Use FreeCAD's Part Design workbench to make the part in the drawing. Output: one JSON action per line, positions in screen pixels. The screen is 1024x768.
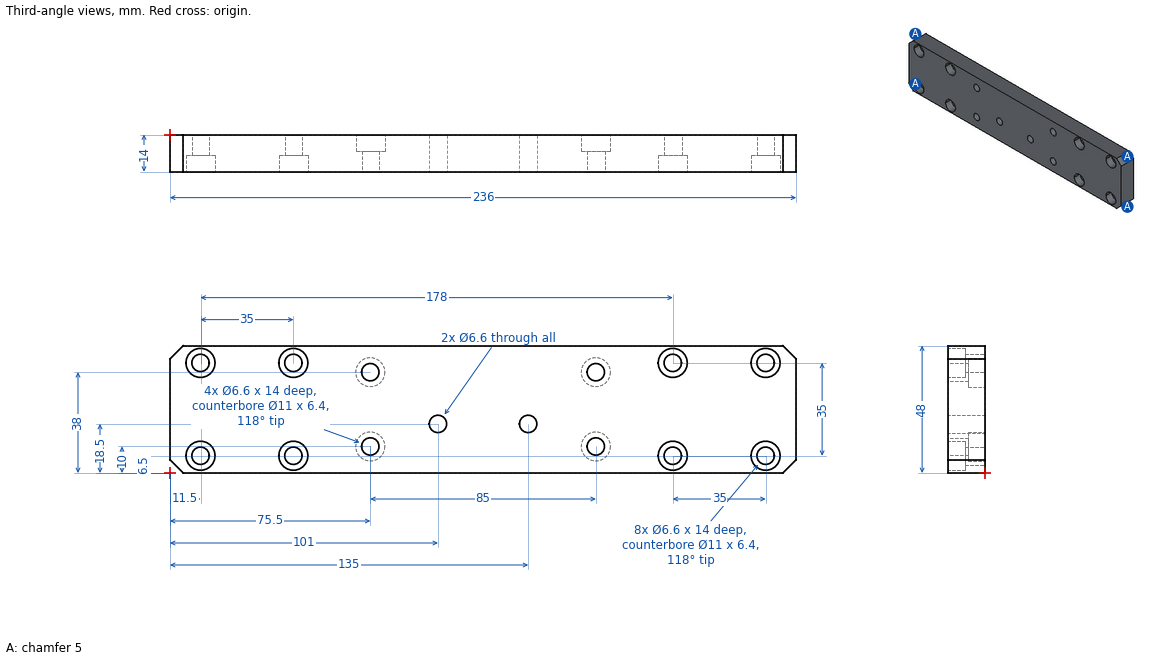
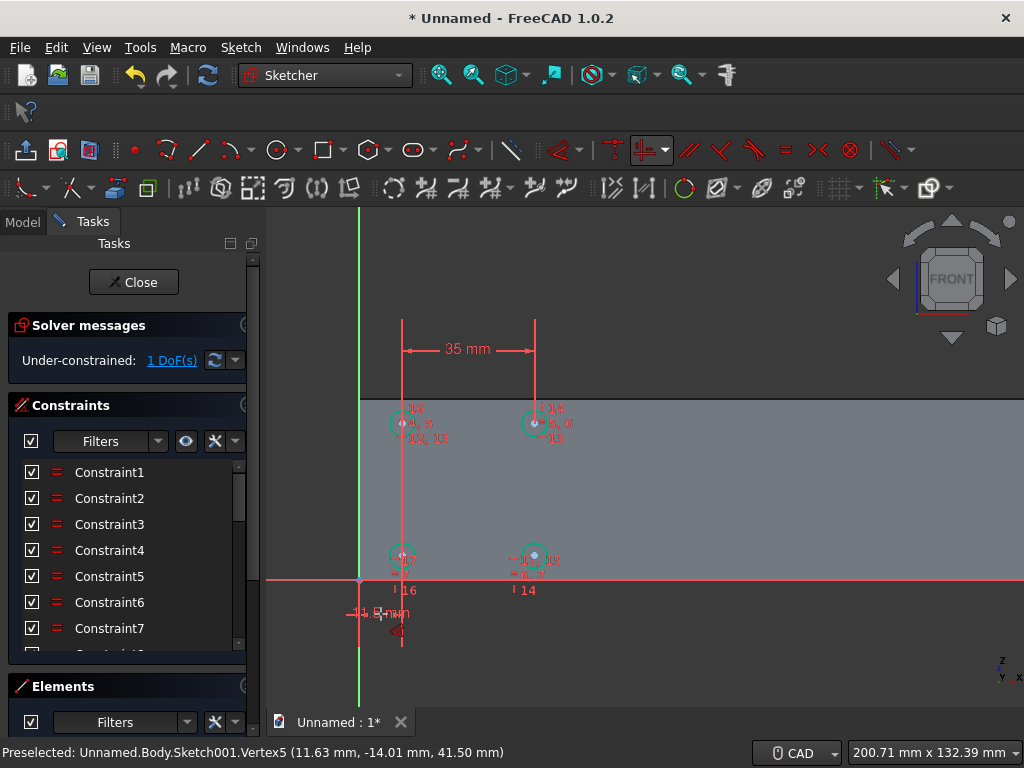
{"action": "scroll", "coordinate": [403, 425], "scroll_direction": "down", "scroll_amount": 4}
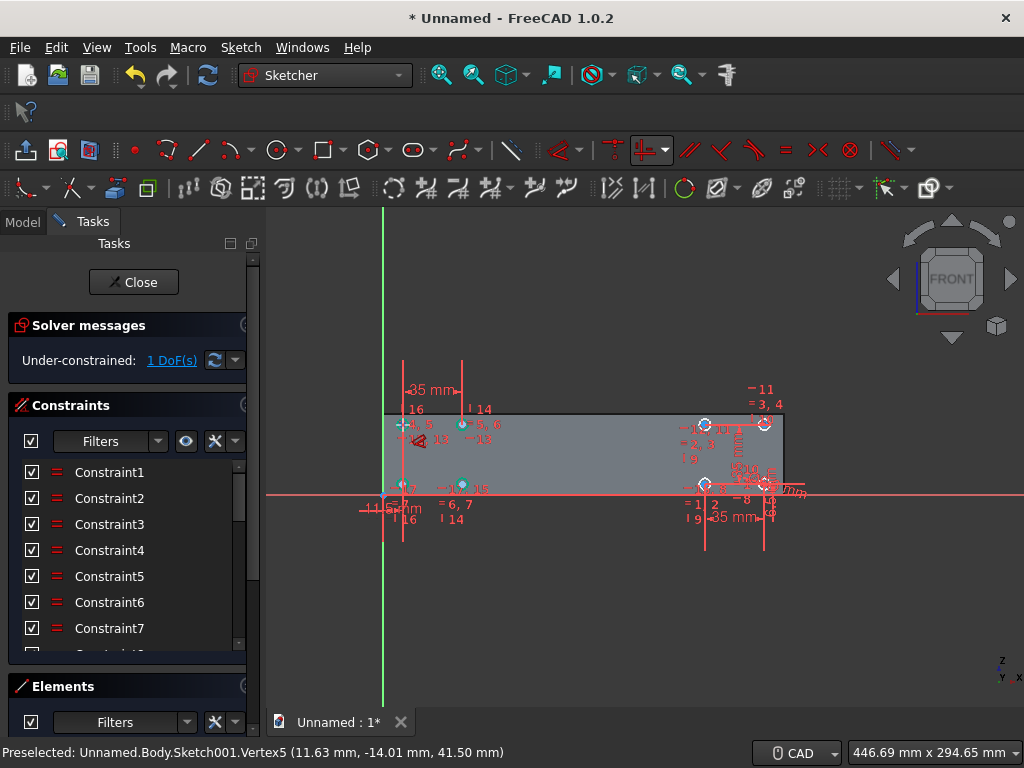
{"action": "left_click", "coordinate": [705, 425]}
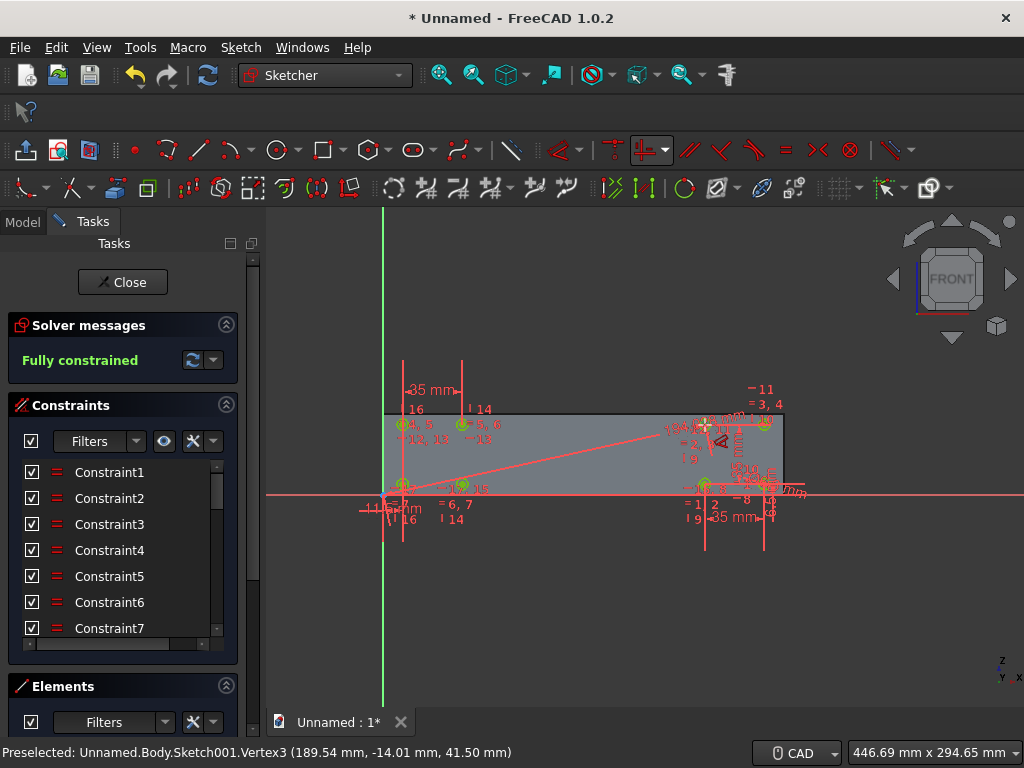
{"action": "left_click", "coordinate": [403, 425]}
{"action": "left_click", "coordinate": [554, 391]}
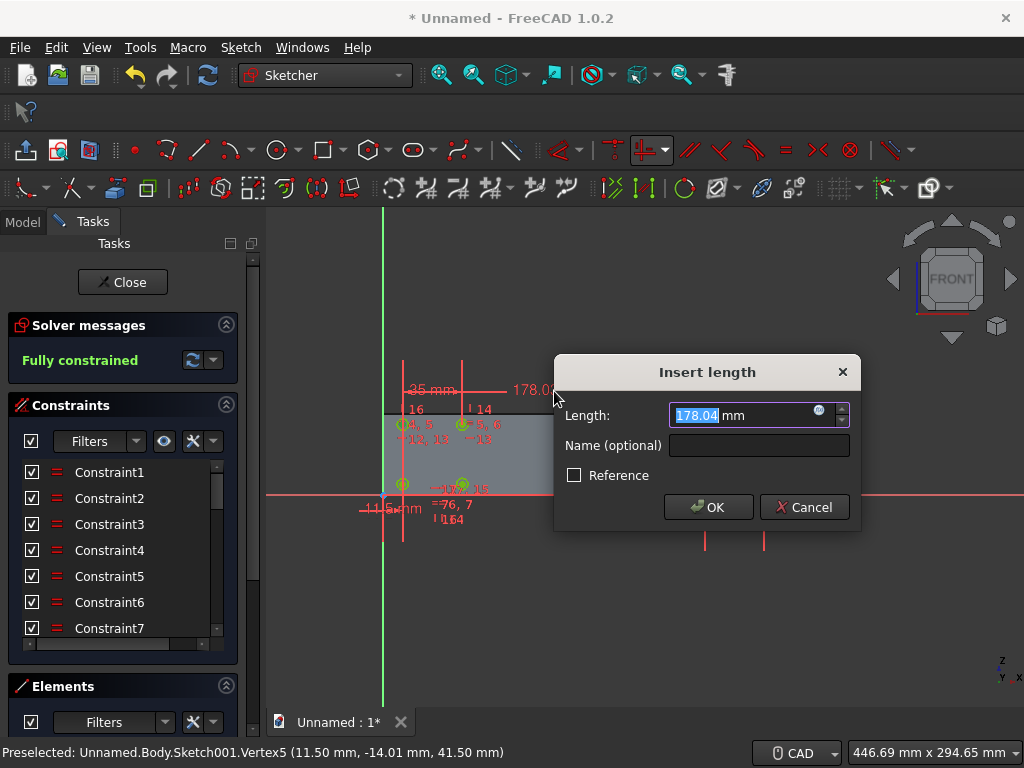
{"action": "type", "text": "178"}
{"action": "key", "text": "Return"}
{"action": "key", "text": "Escape"}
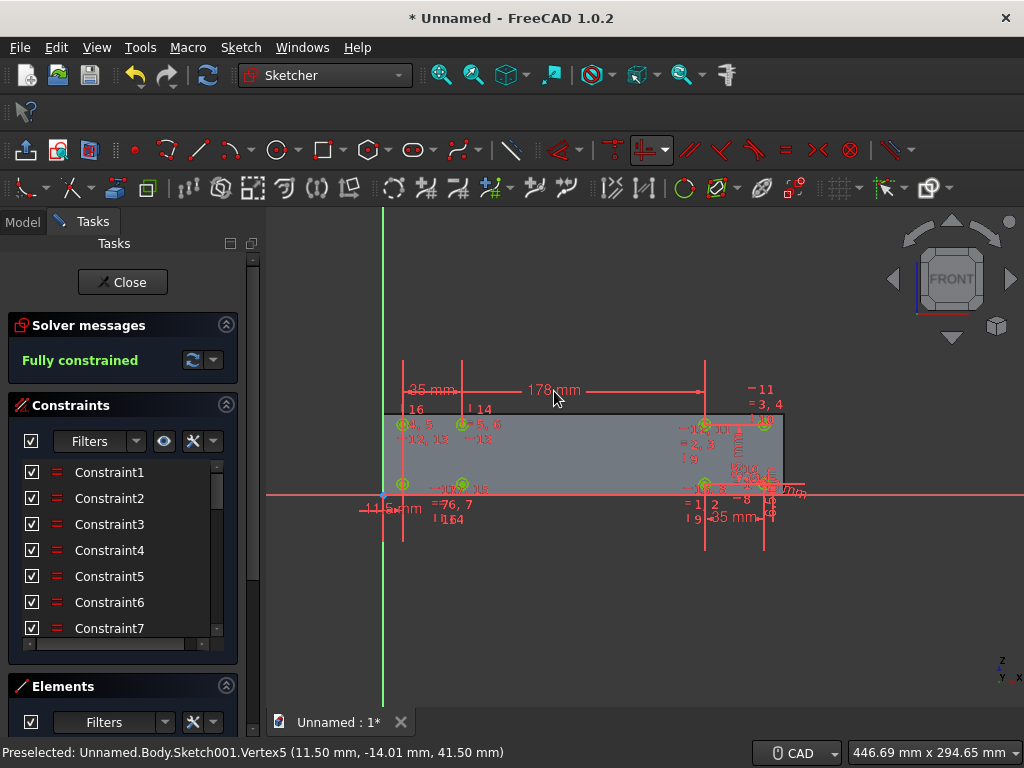
{"action": "left_click", "coordinate": [123, 282]}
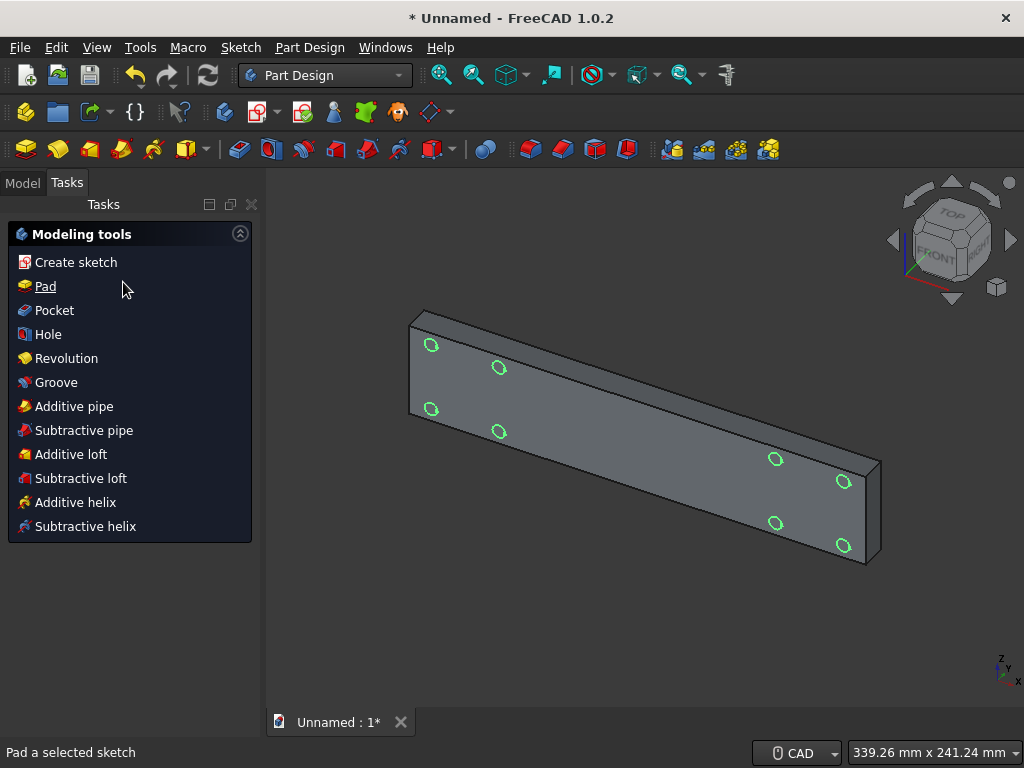
{"action": "left_click", "coordinate": [272, 150]}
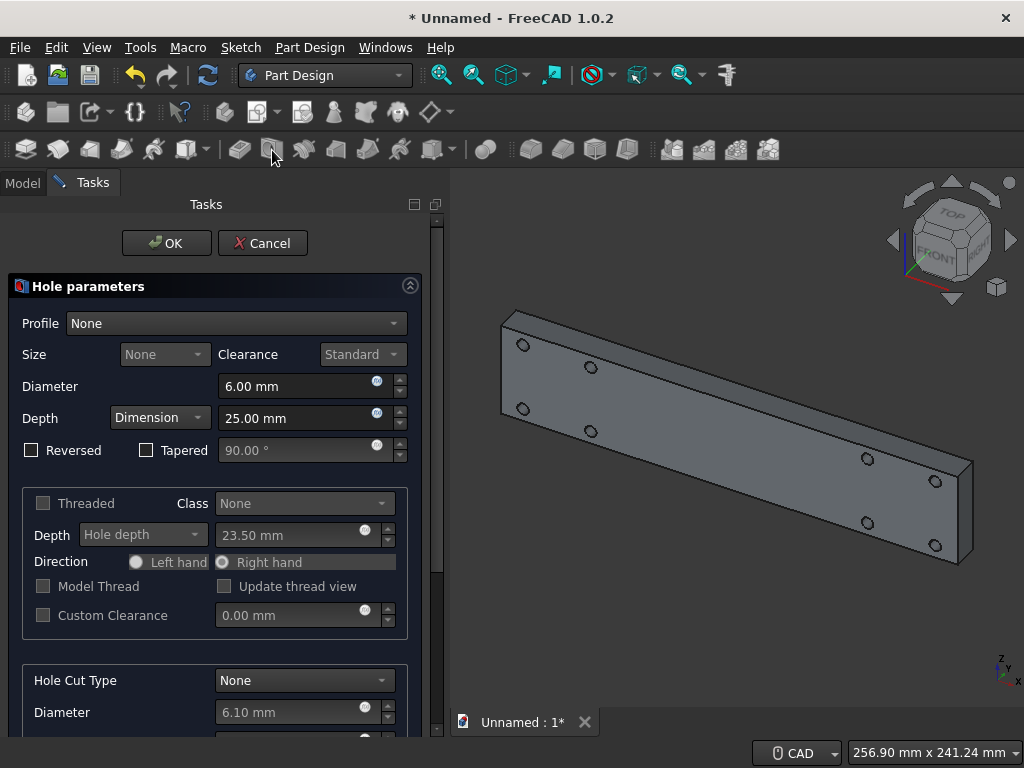
{"action": "triple_click", "coordinate": [305, 386]}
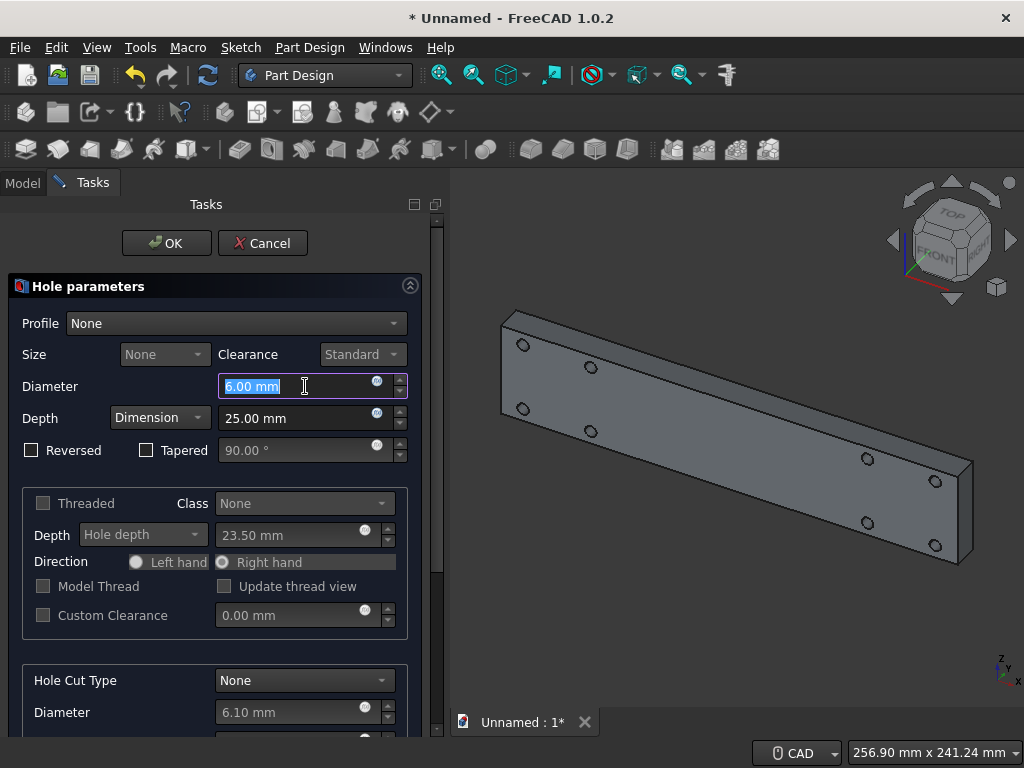
{"action": "type", "text": "6.6"}
{"action": "key", "text": "Tab"}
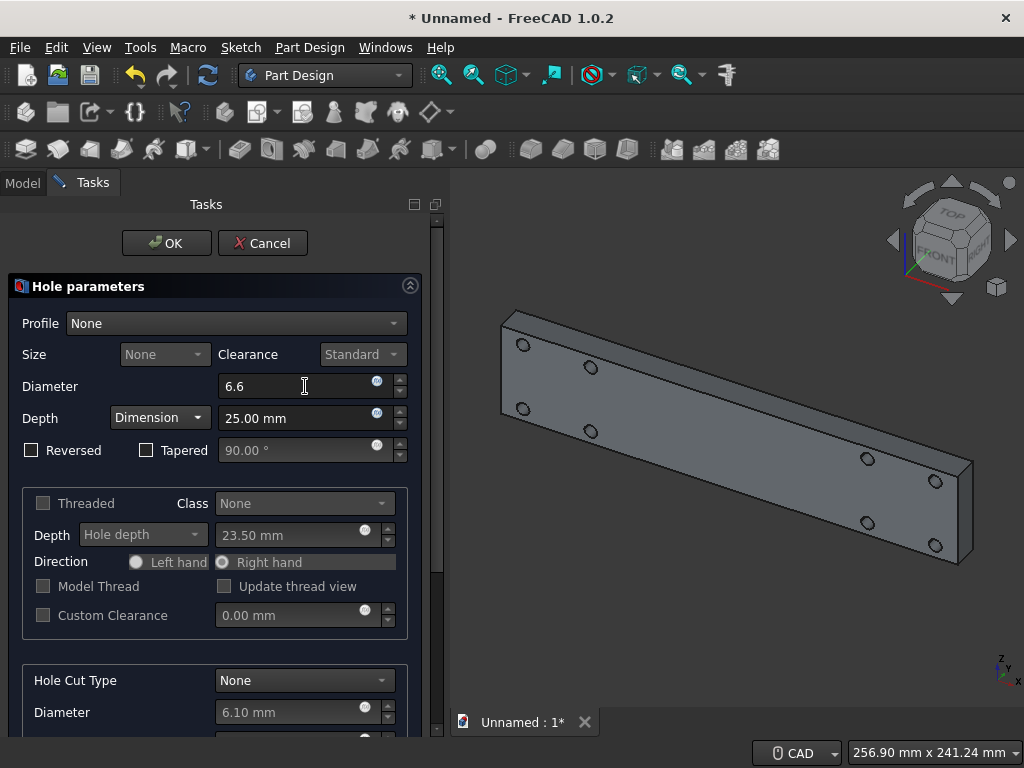
{"action": "triple_click", "coordinate": [305, 418]}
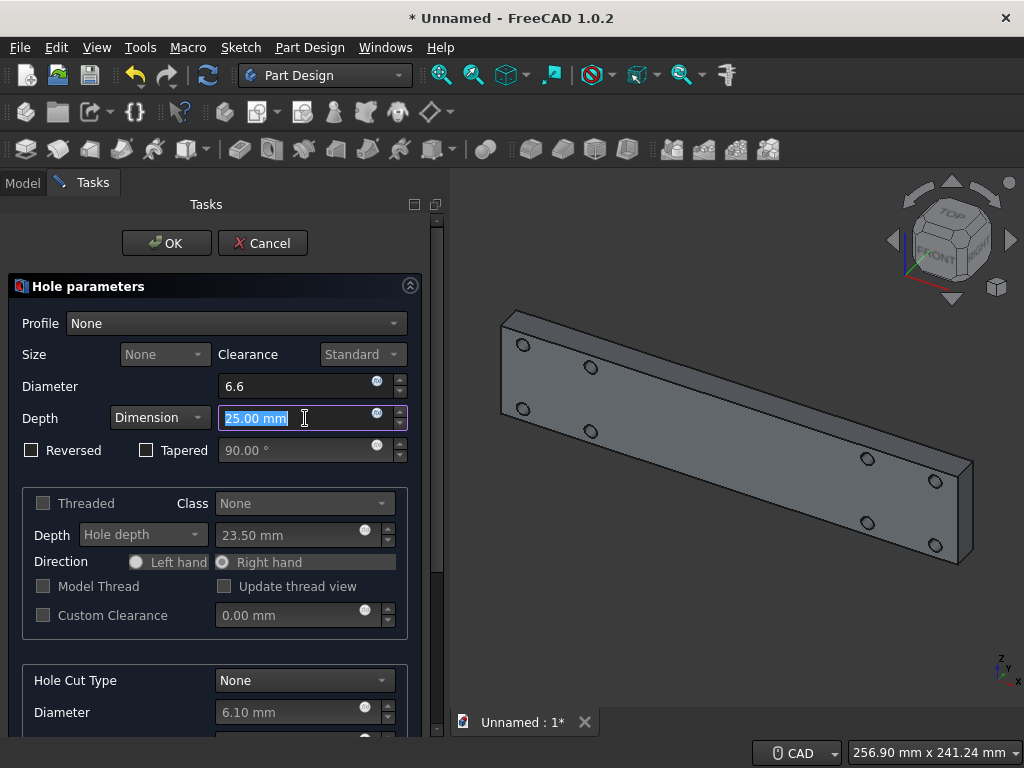
{"action": "type", "text": "14"}
{"action": "key", "text": "Tab"}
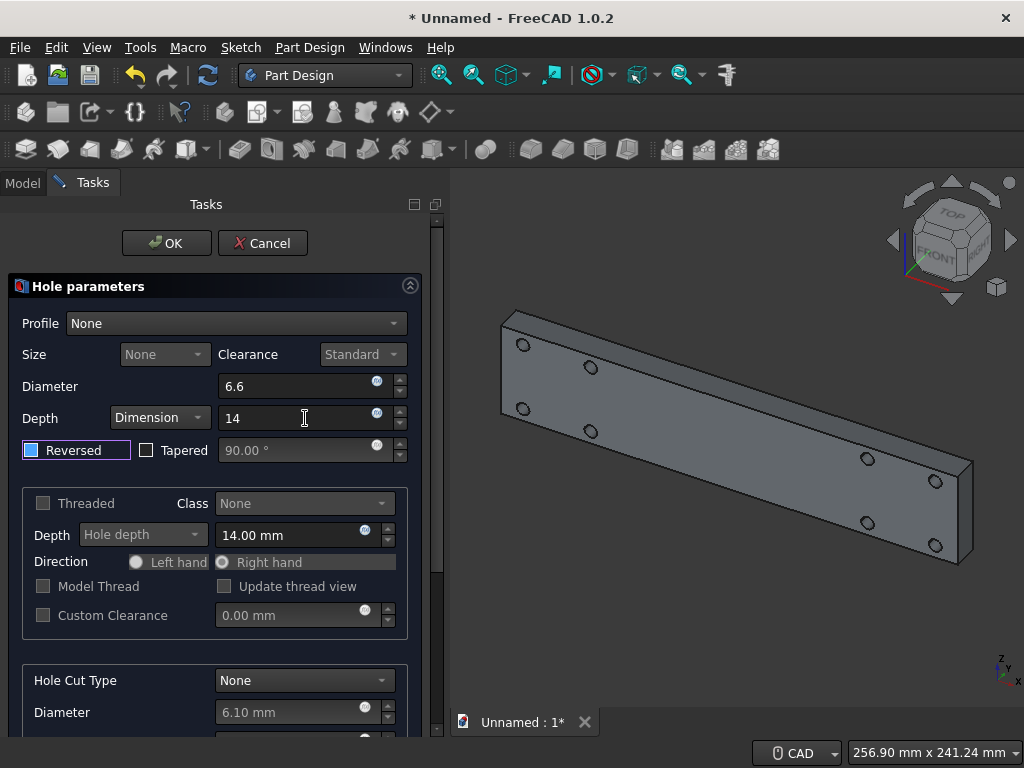
{"action": "left_click", "coordinate": [306, 680]}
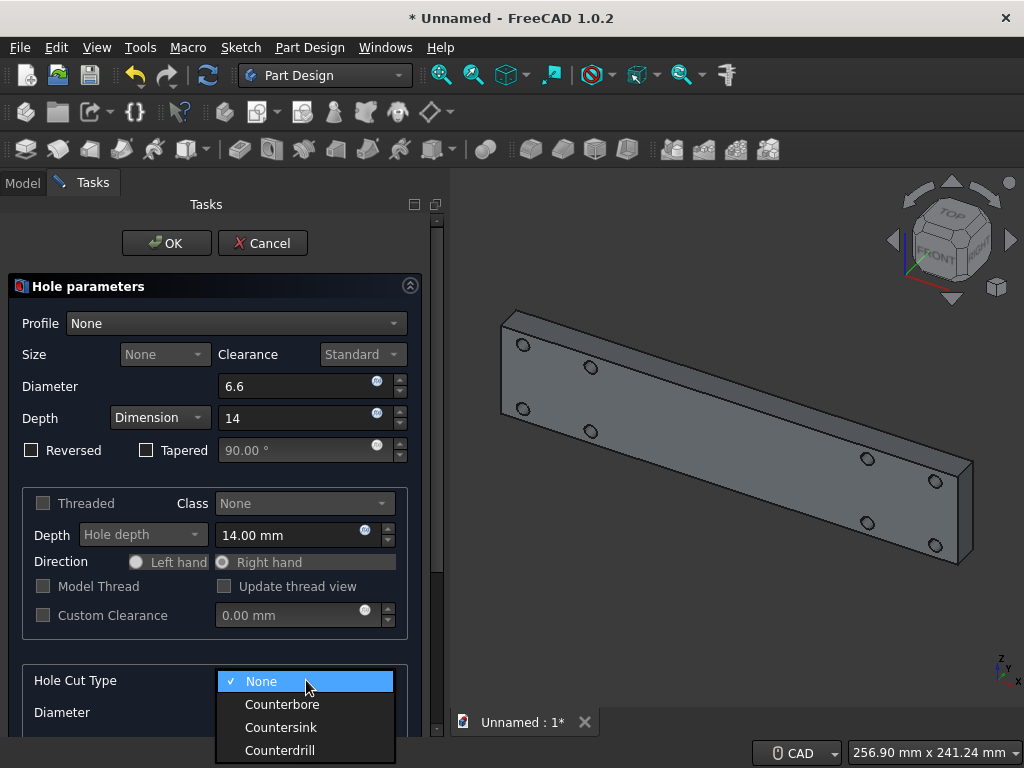
{"action": "left_click", "coordinate": [304, 704]}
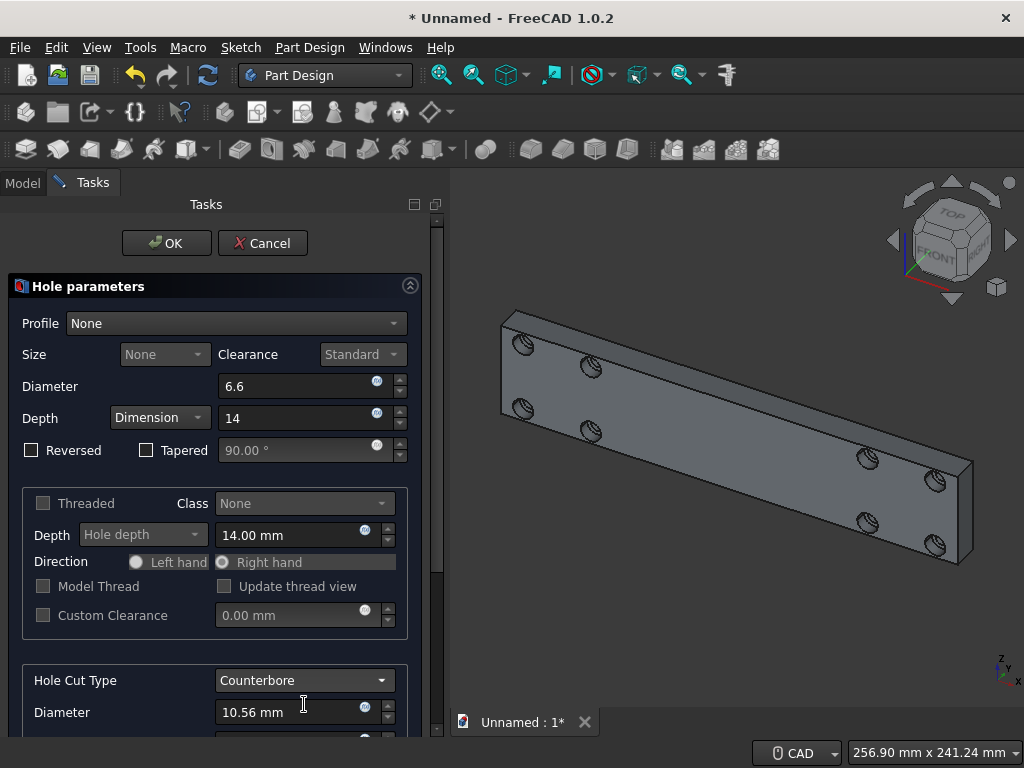
{"action": "triple_click", "coordinate": [298, 712]}